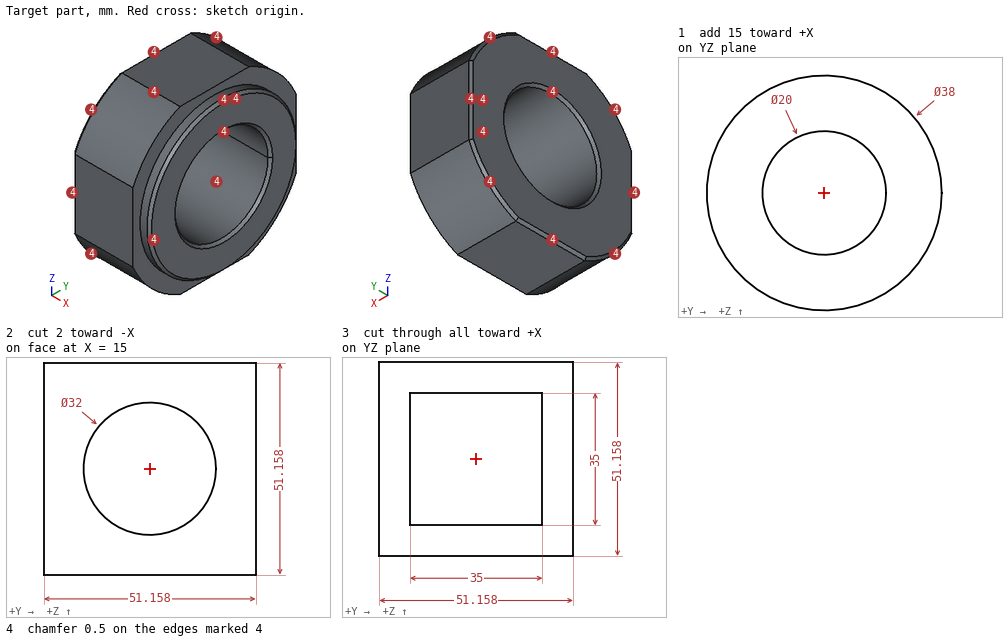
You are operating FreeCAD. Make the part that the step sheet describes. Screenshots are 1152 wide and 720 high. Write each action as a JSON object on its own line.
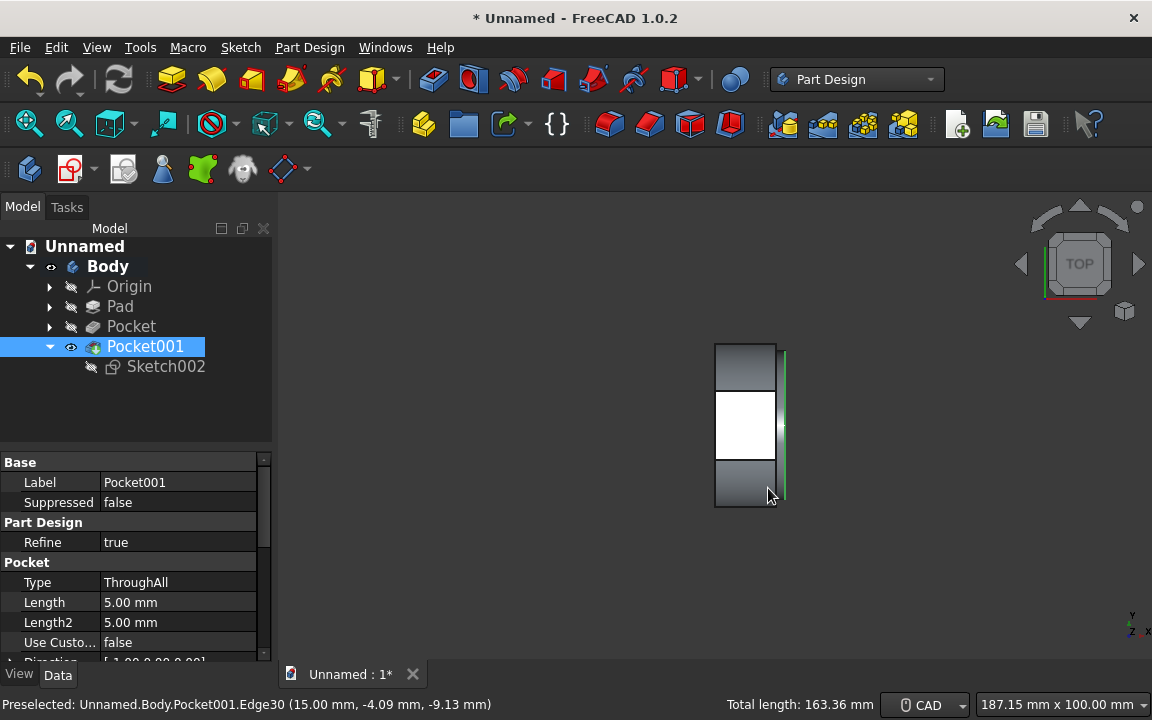
{"action": "left_click", "coordinate": [30, 124]}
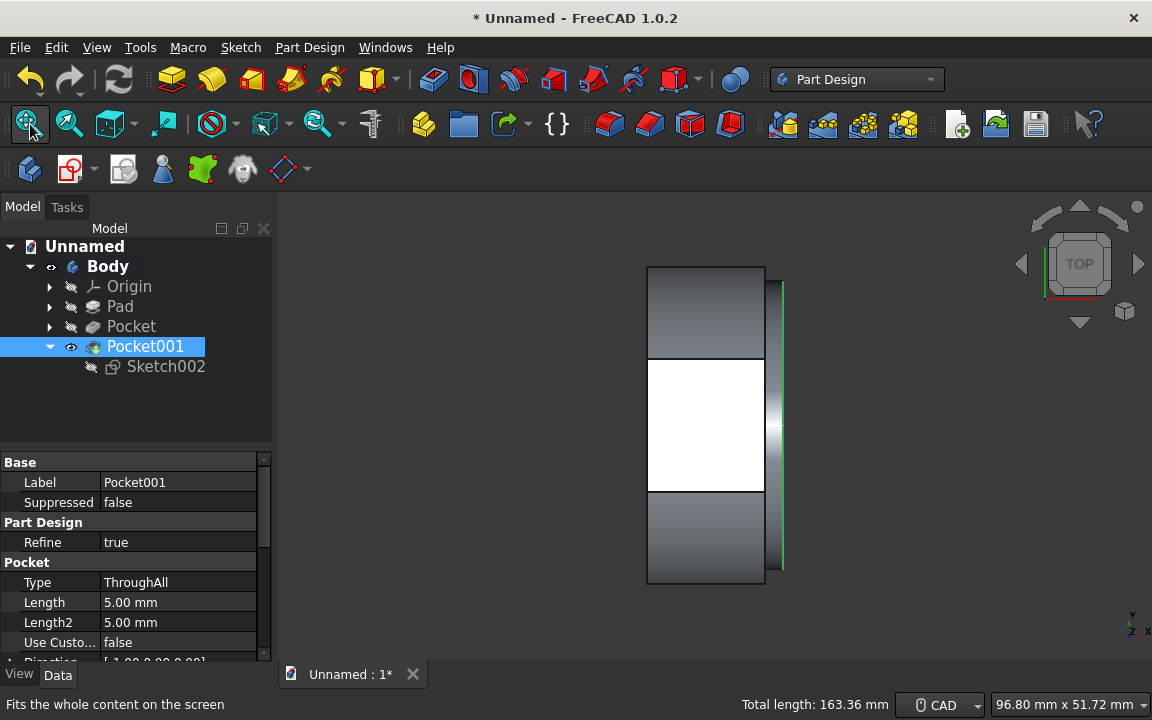
{"action": "key", "text": "1"}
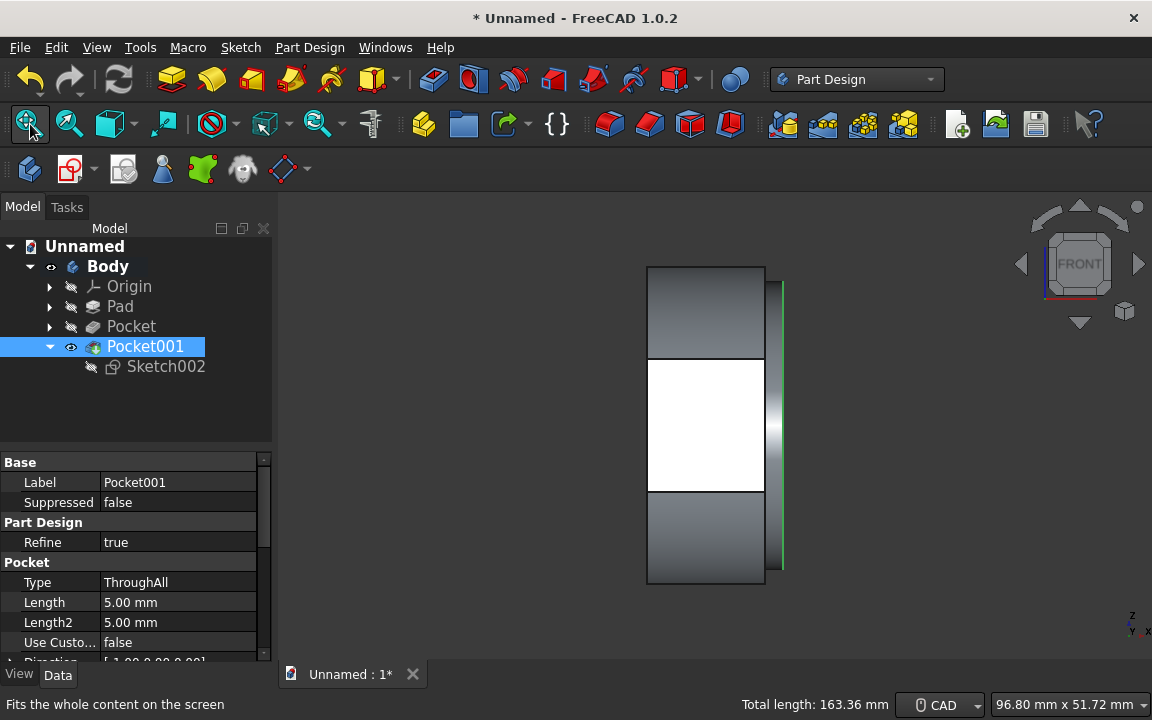
{"action": "key", "text": "3"}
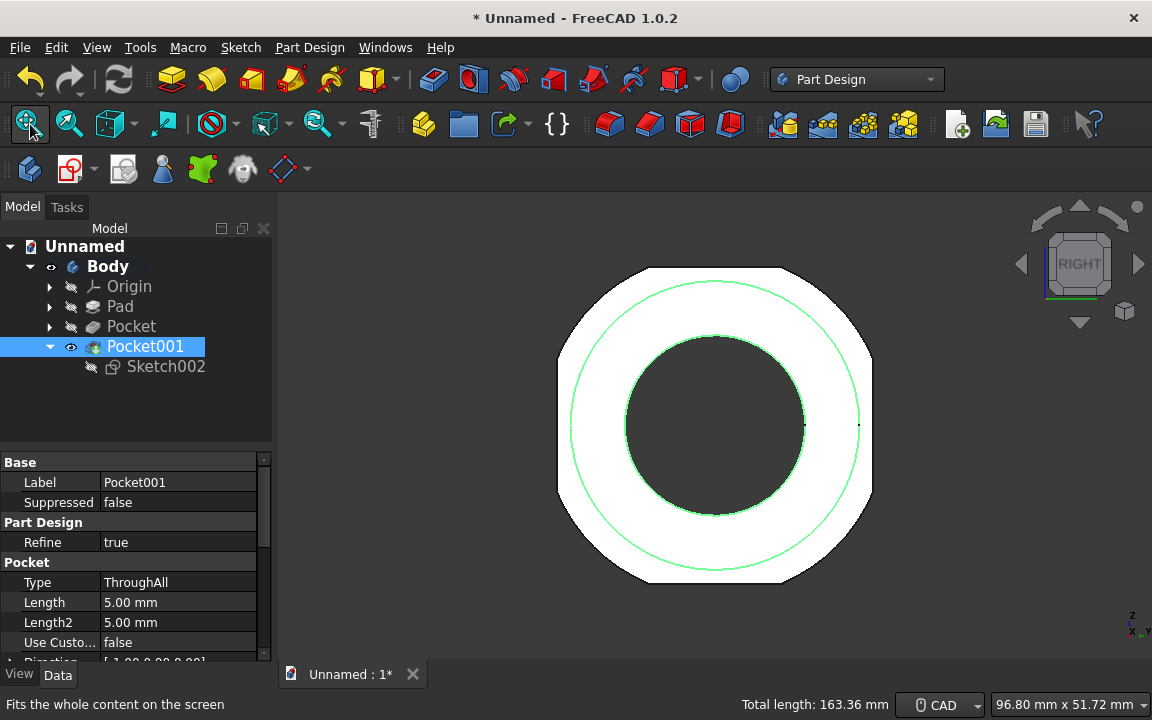
{"action": "key", "text": "5"}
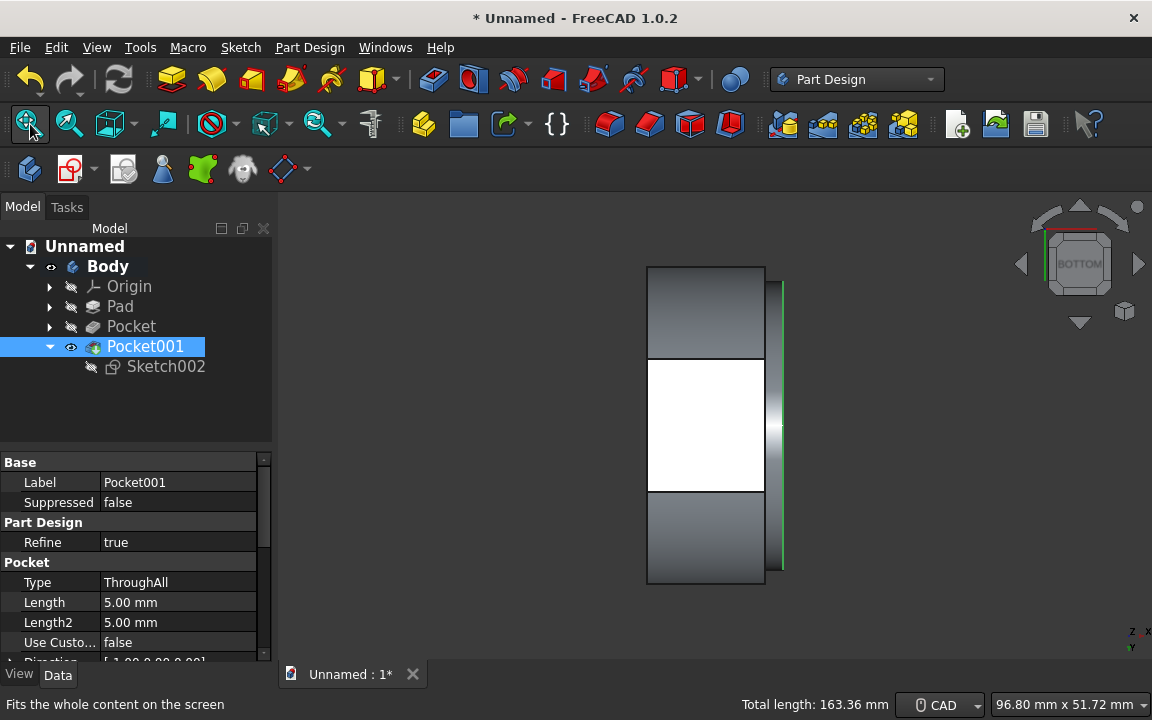
{"action": "key", "text": "4"}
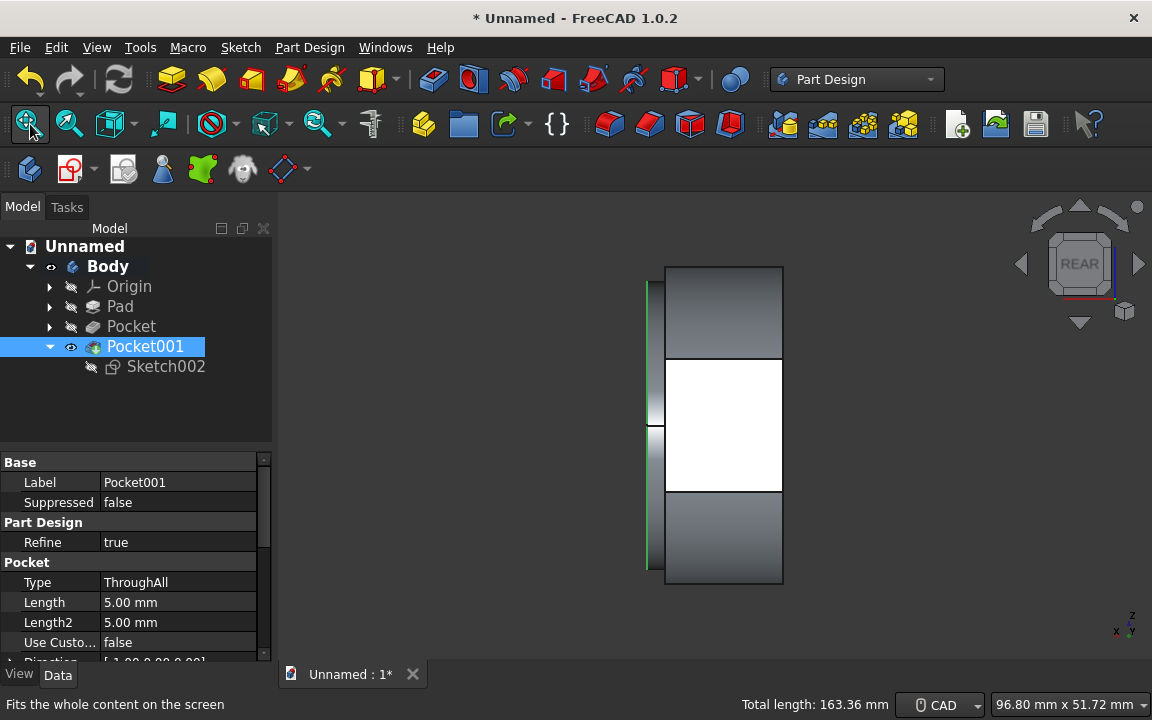
{"action": "key", "text": "6"}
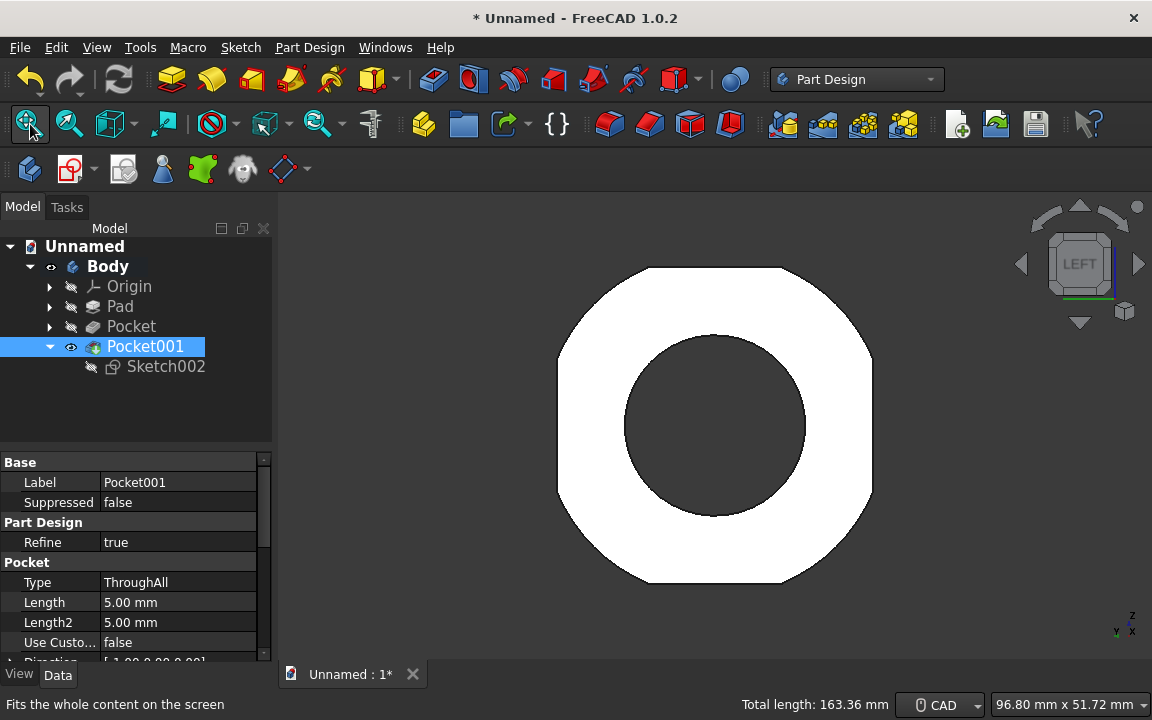
{"action": "left_click", "coordinate": [625, 515], "text": "ctrl"}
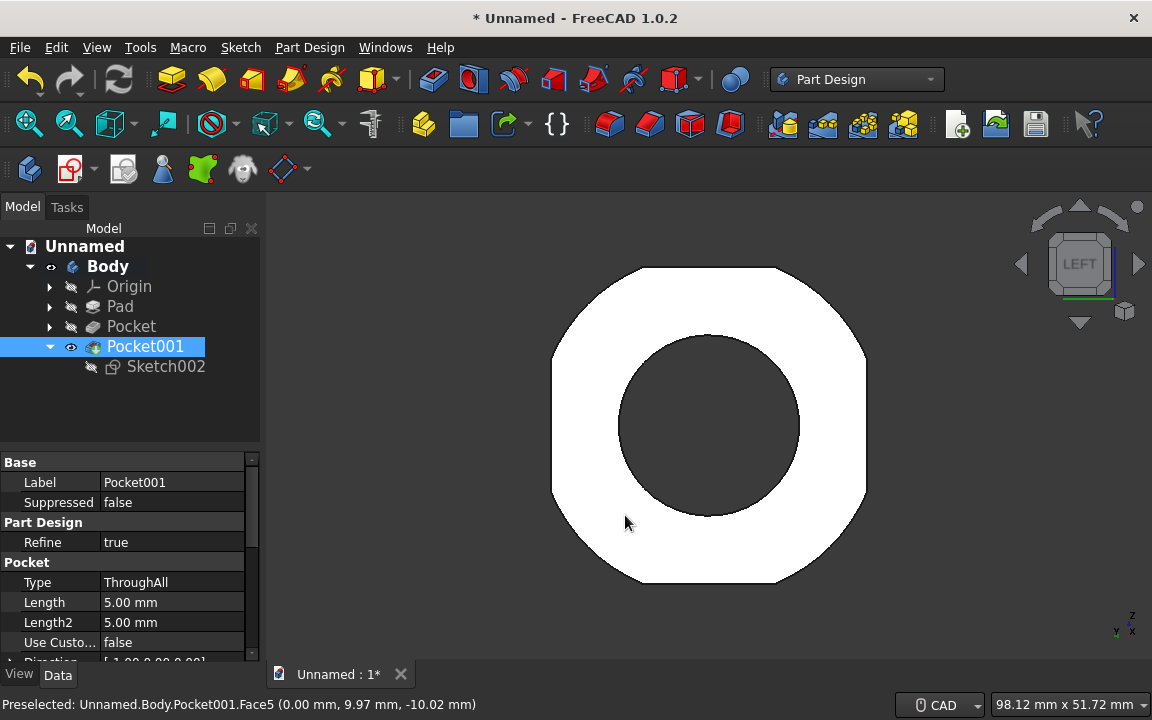
{"action": "left_click", "coordinate": [650, 124]}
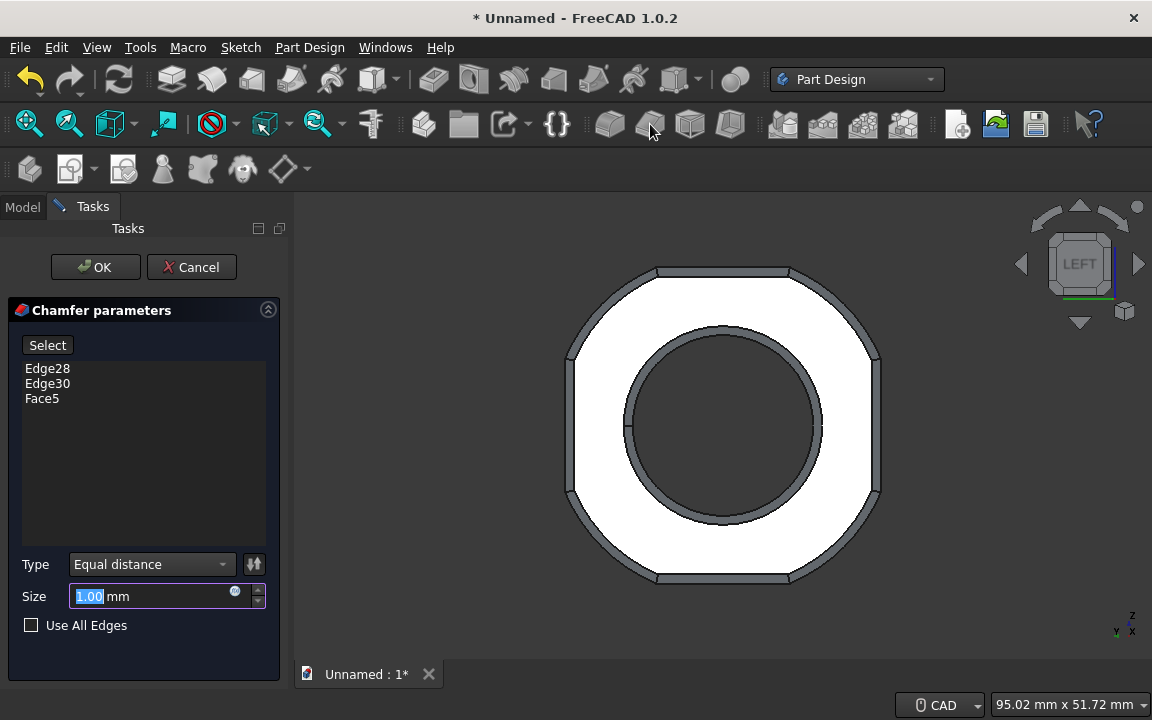
{"action": "type", "text": "0.5"}
{"action": "key", "text": "Tab"}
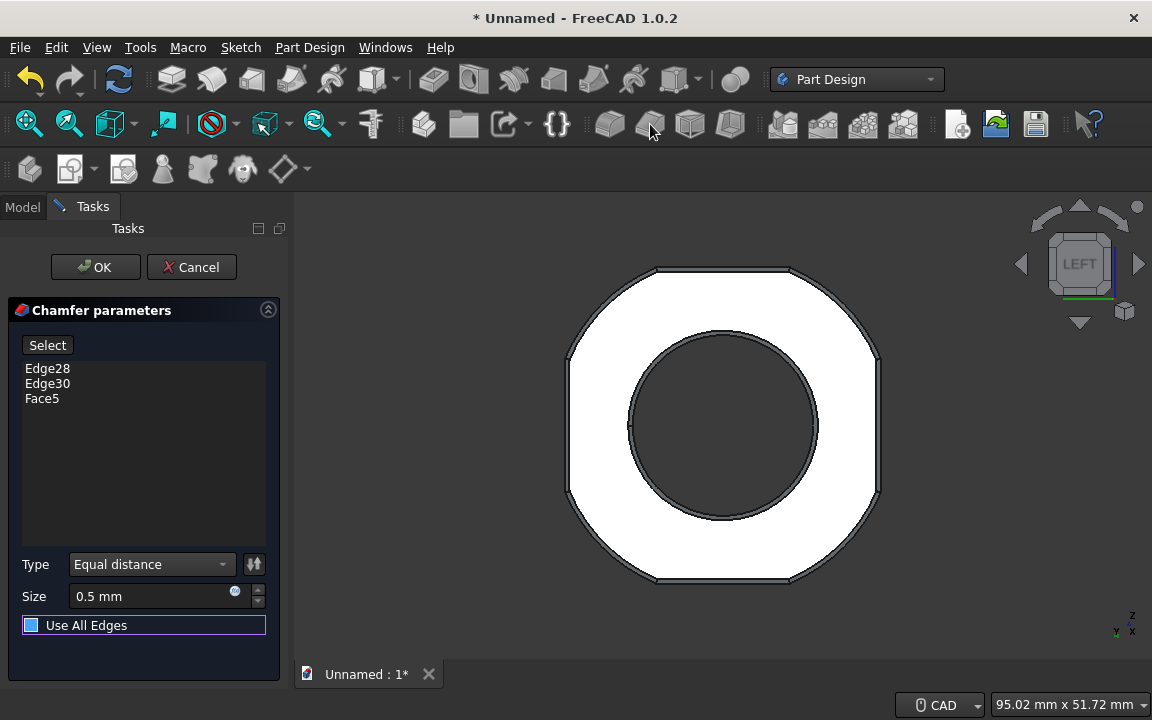
{"action": "left_click", "coordinate": [96, 267]}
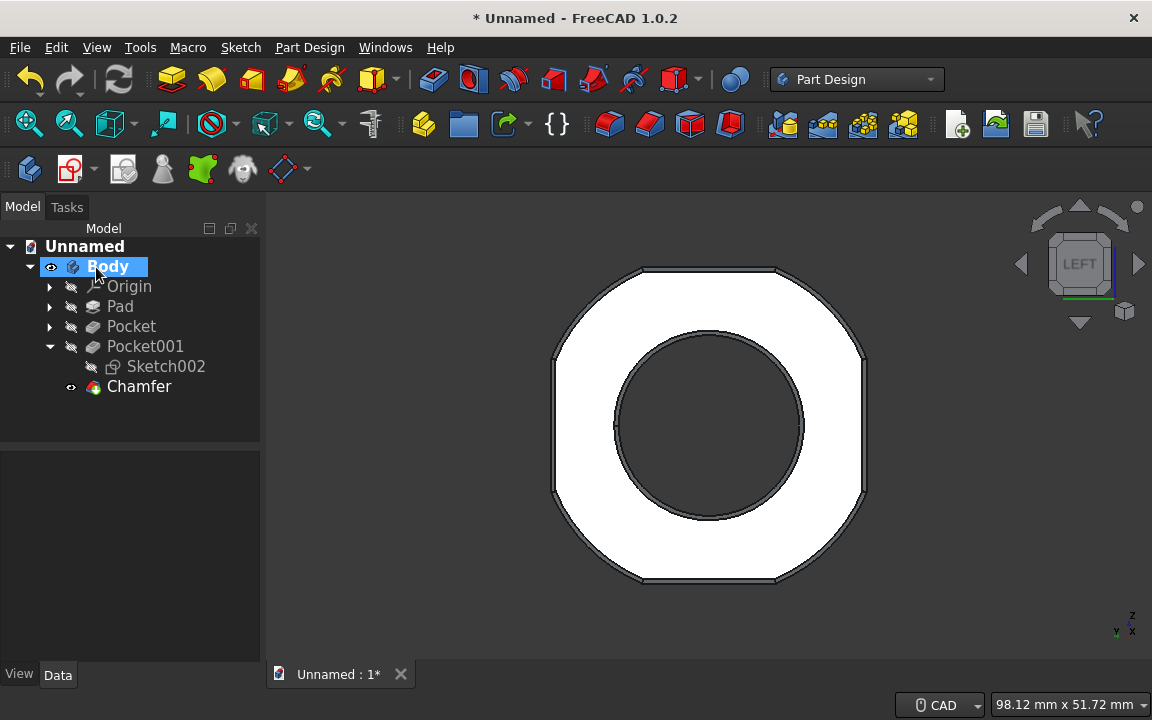
{"action": "key", "text": "0"}